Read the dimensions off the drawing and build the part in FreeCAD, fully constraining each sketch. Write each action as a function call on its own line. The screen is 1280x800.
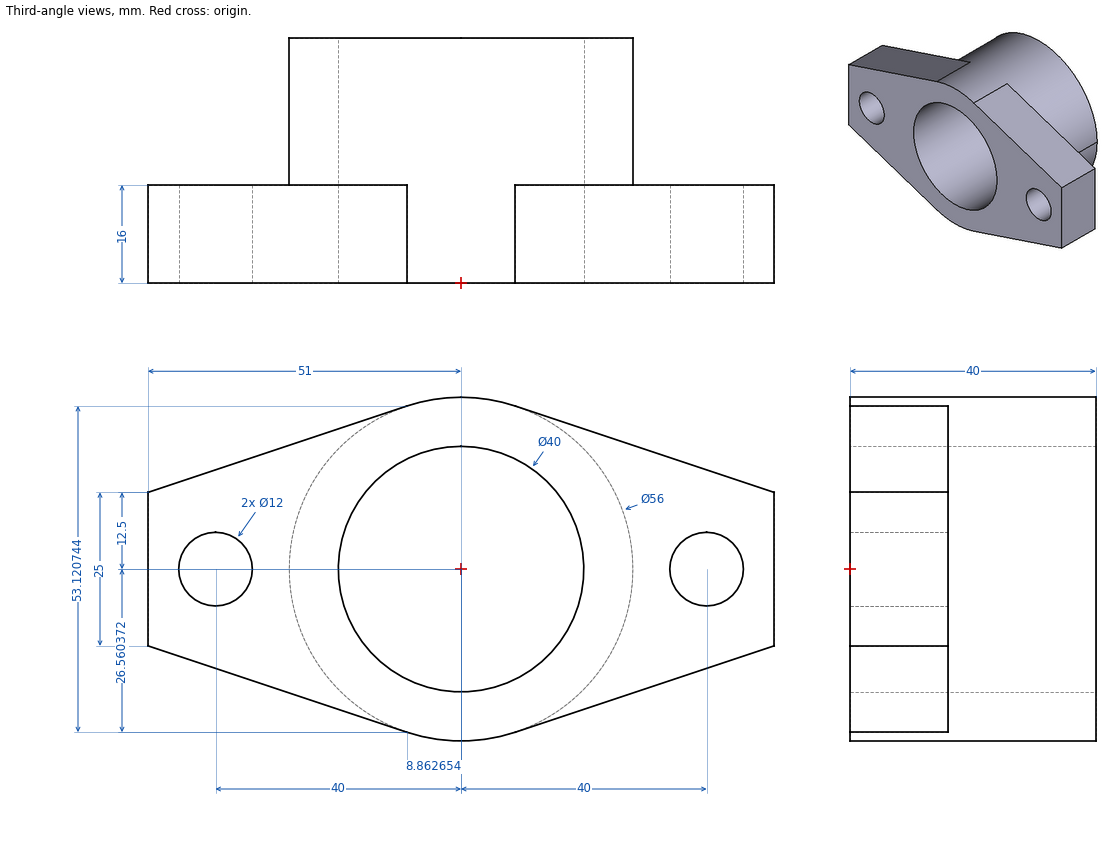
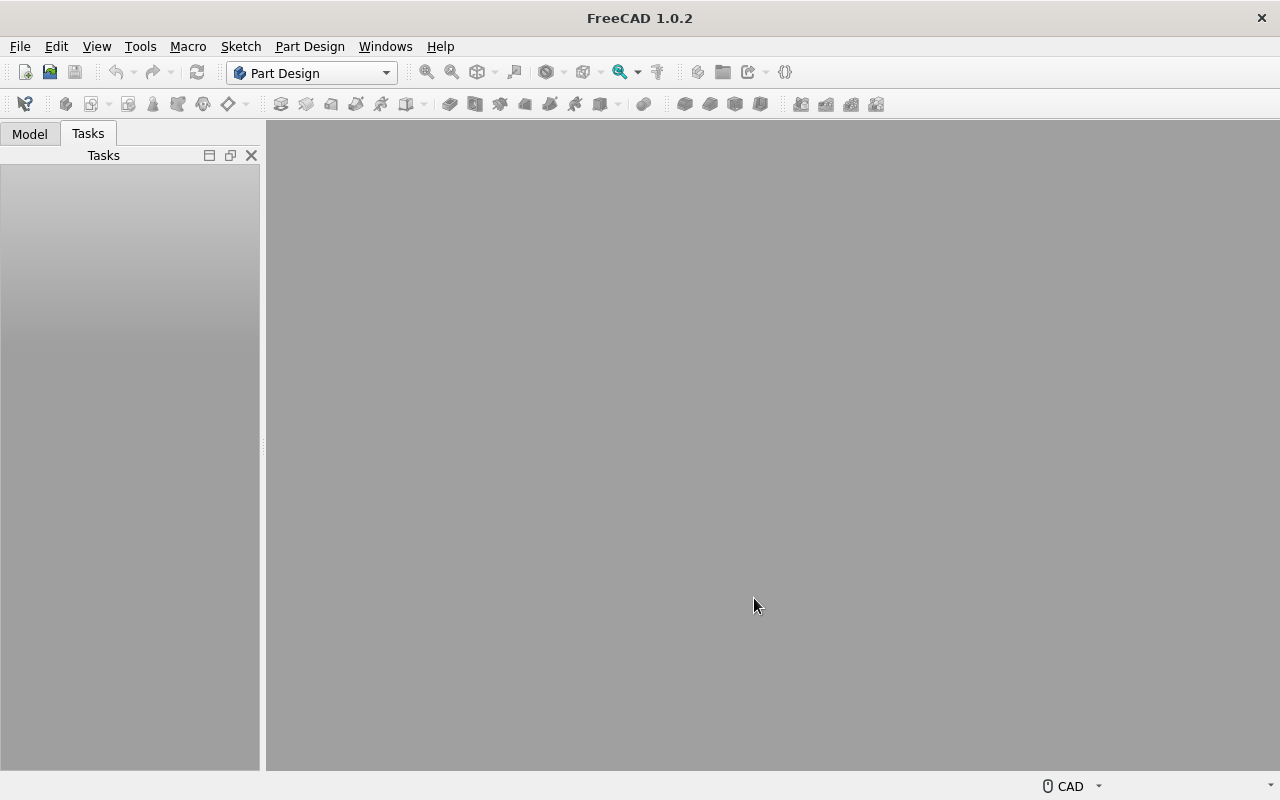
click(25, 72)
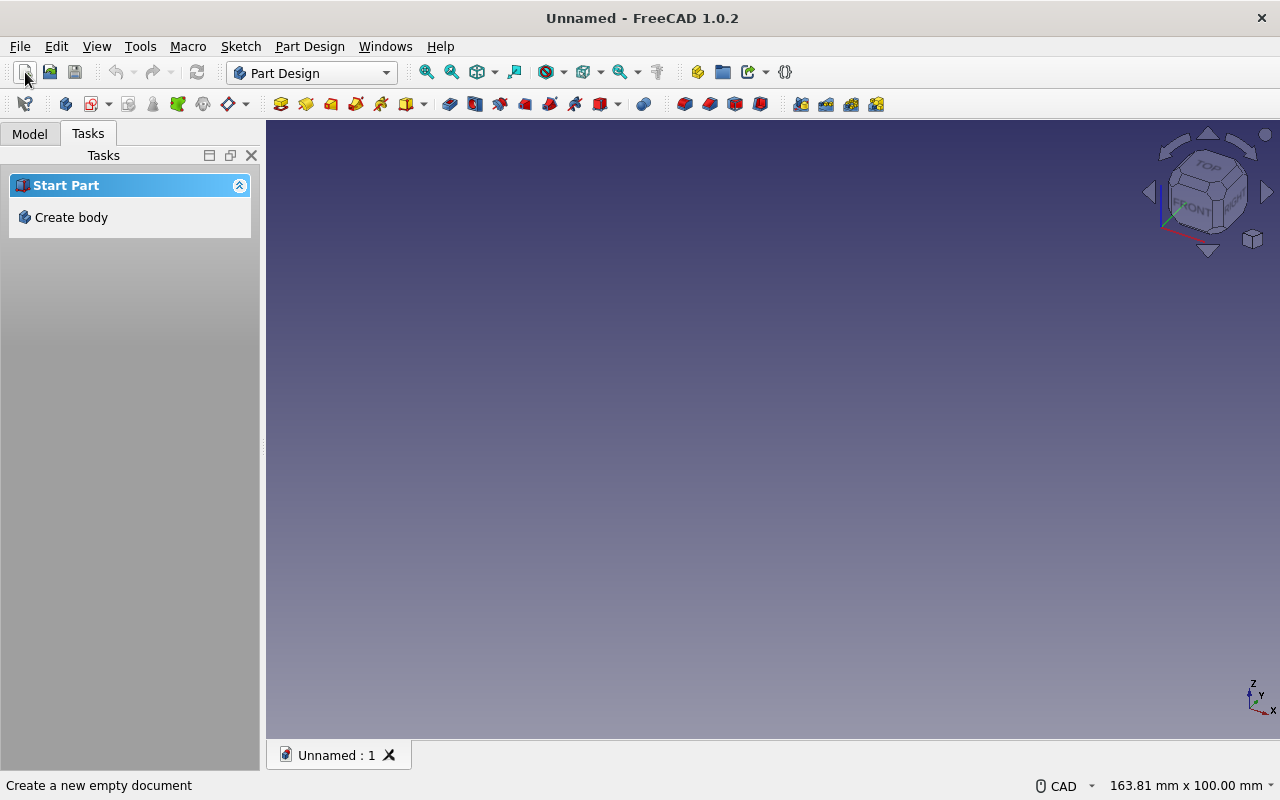
click(90, 104)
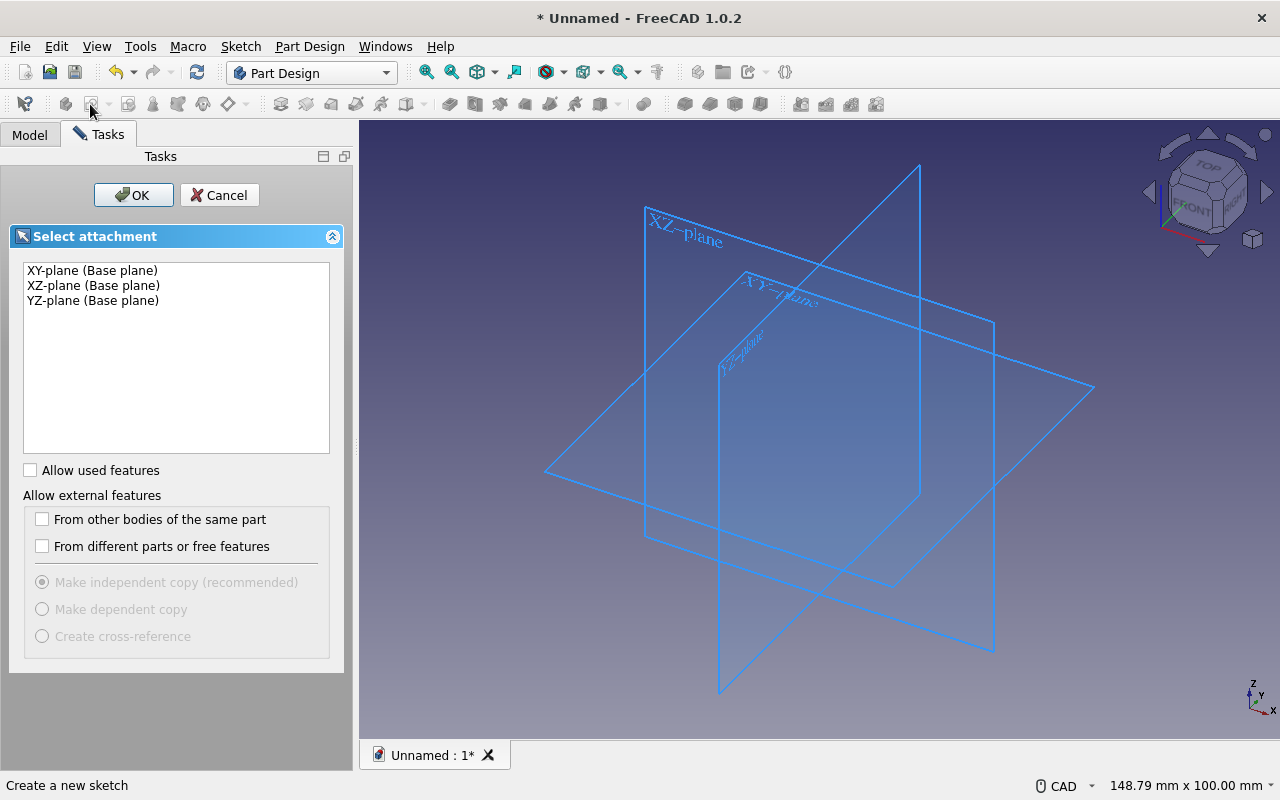
click(84, 286)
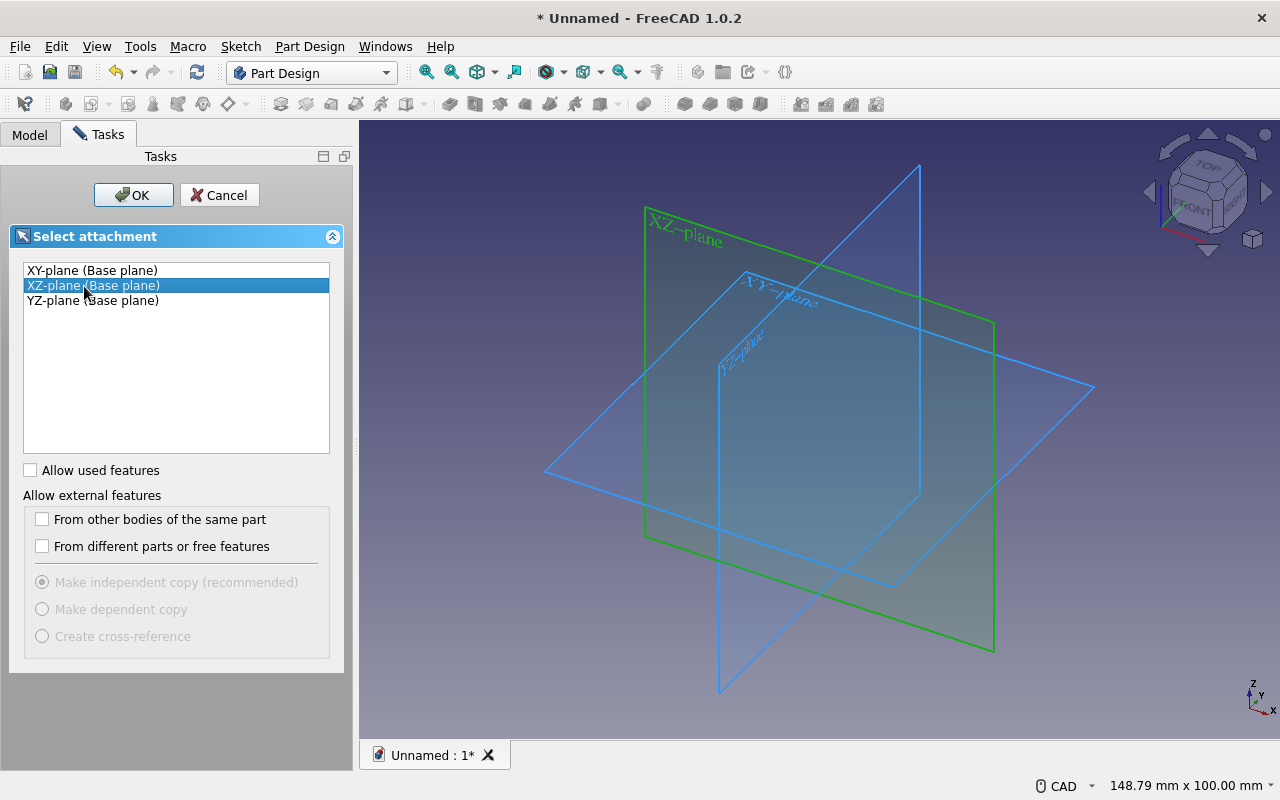
click(134, 195)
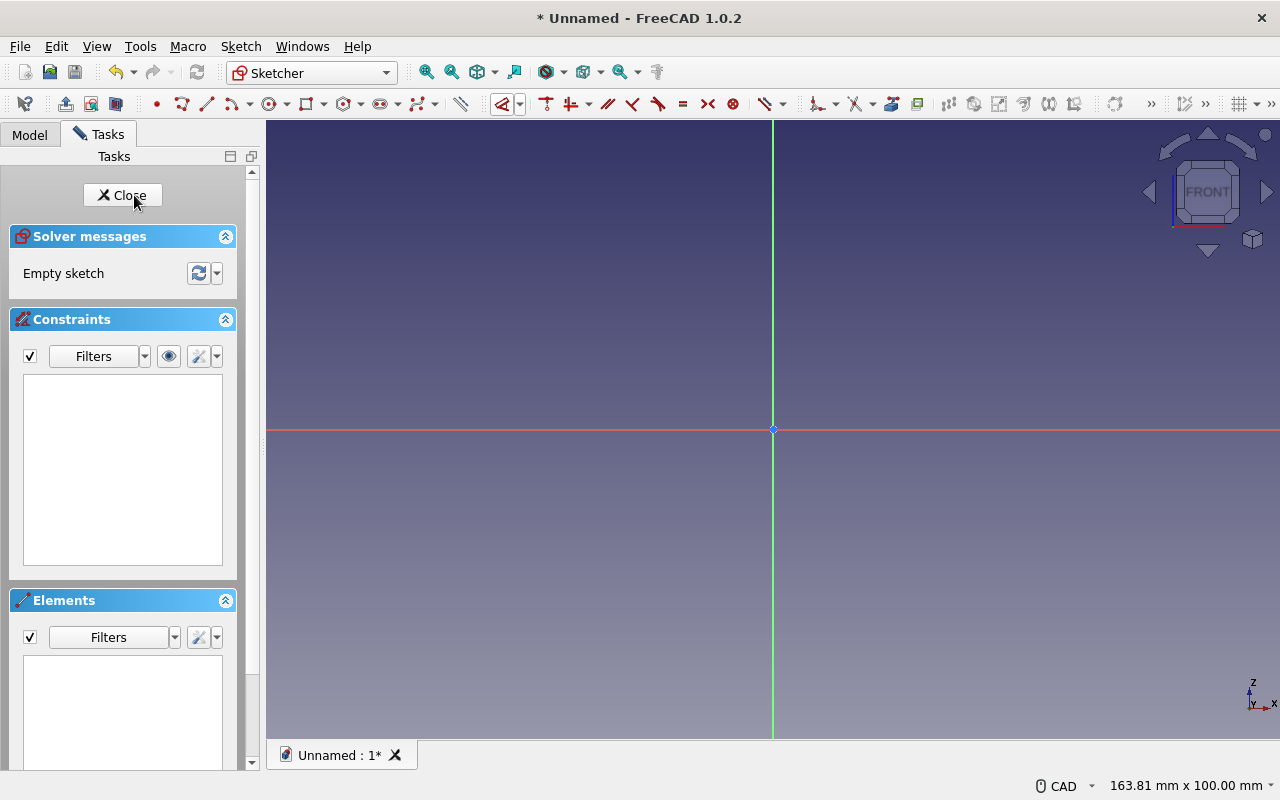
click(268, 104)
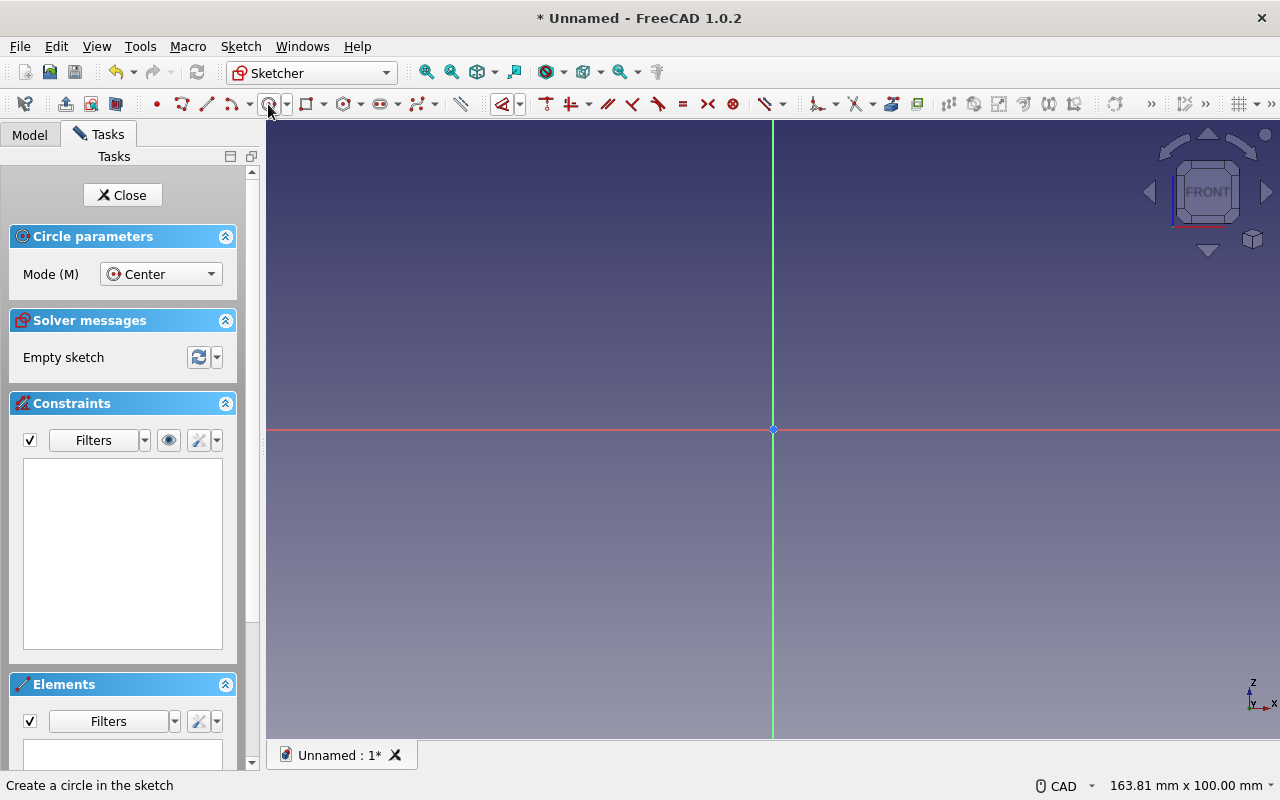
click(773, 430)
move(896, 307)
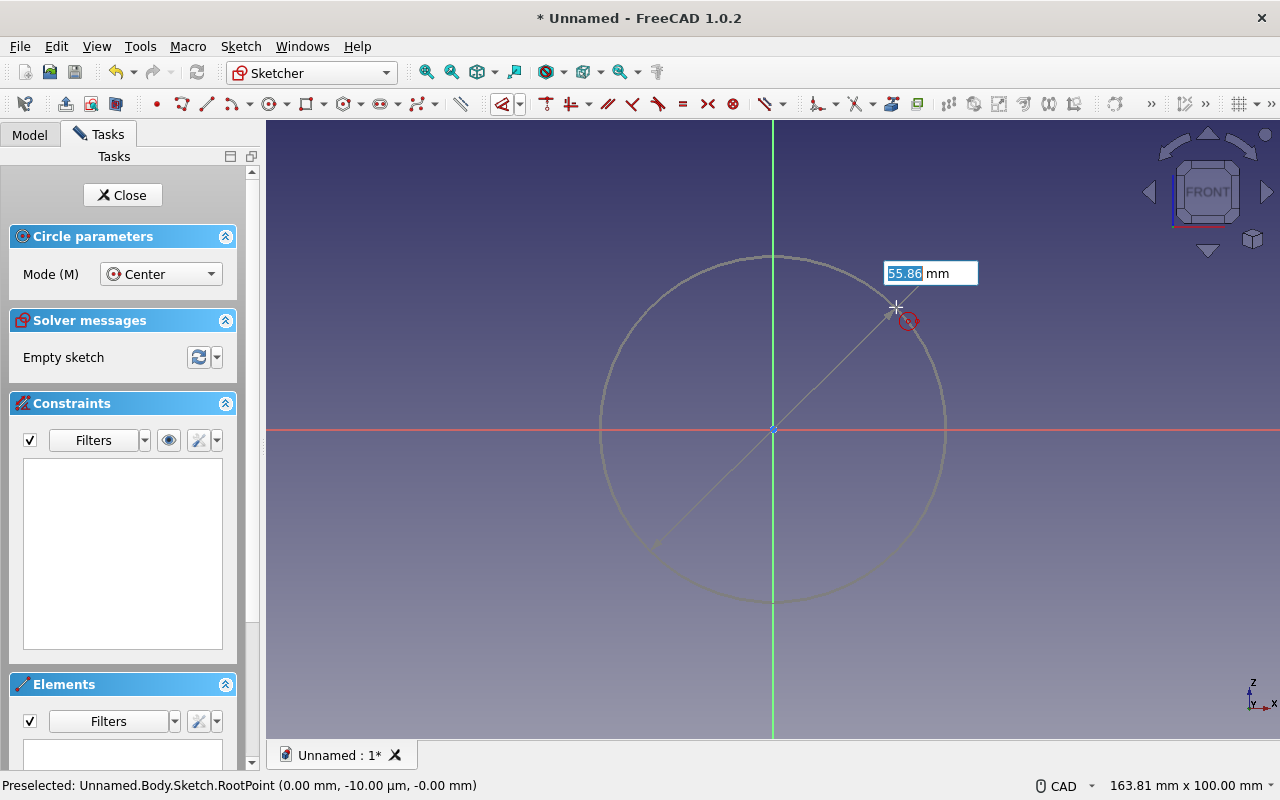
text(56)
key(Return)
key(Escape)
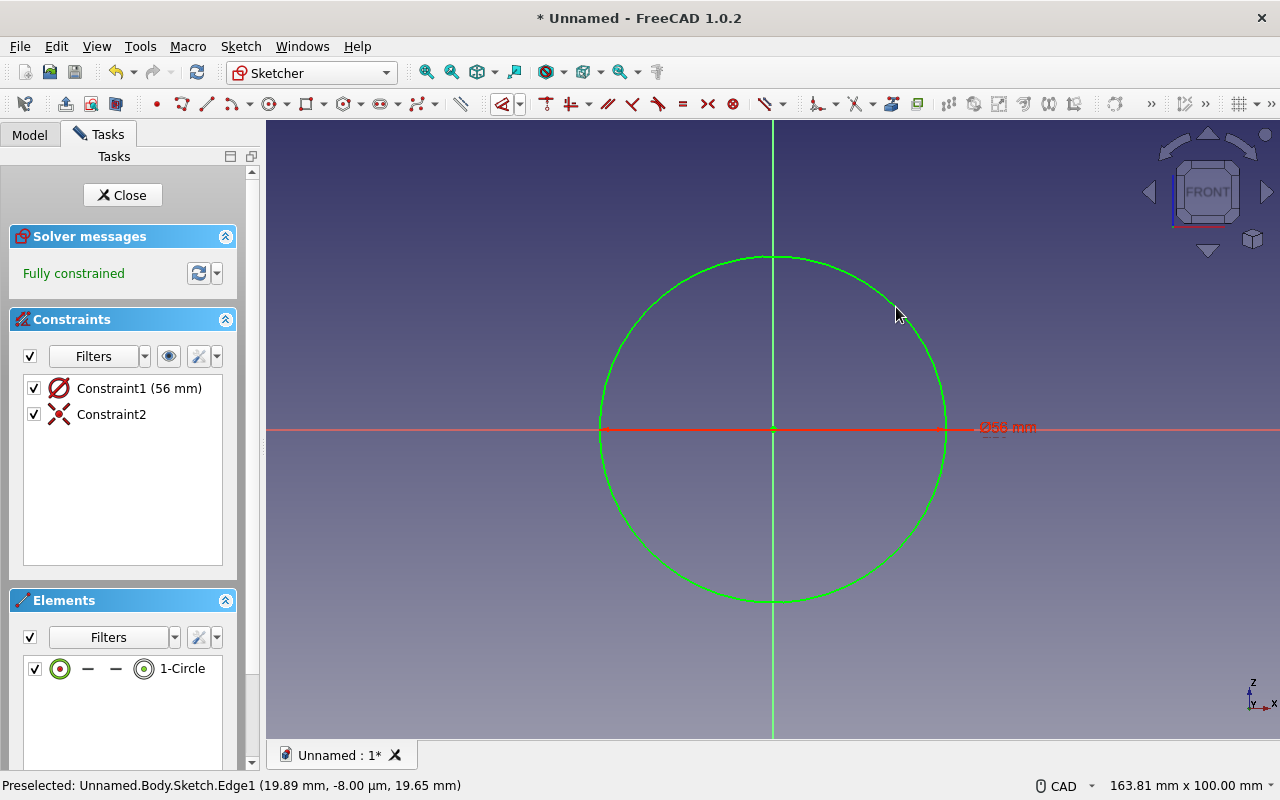
click(123, 195)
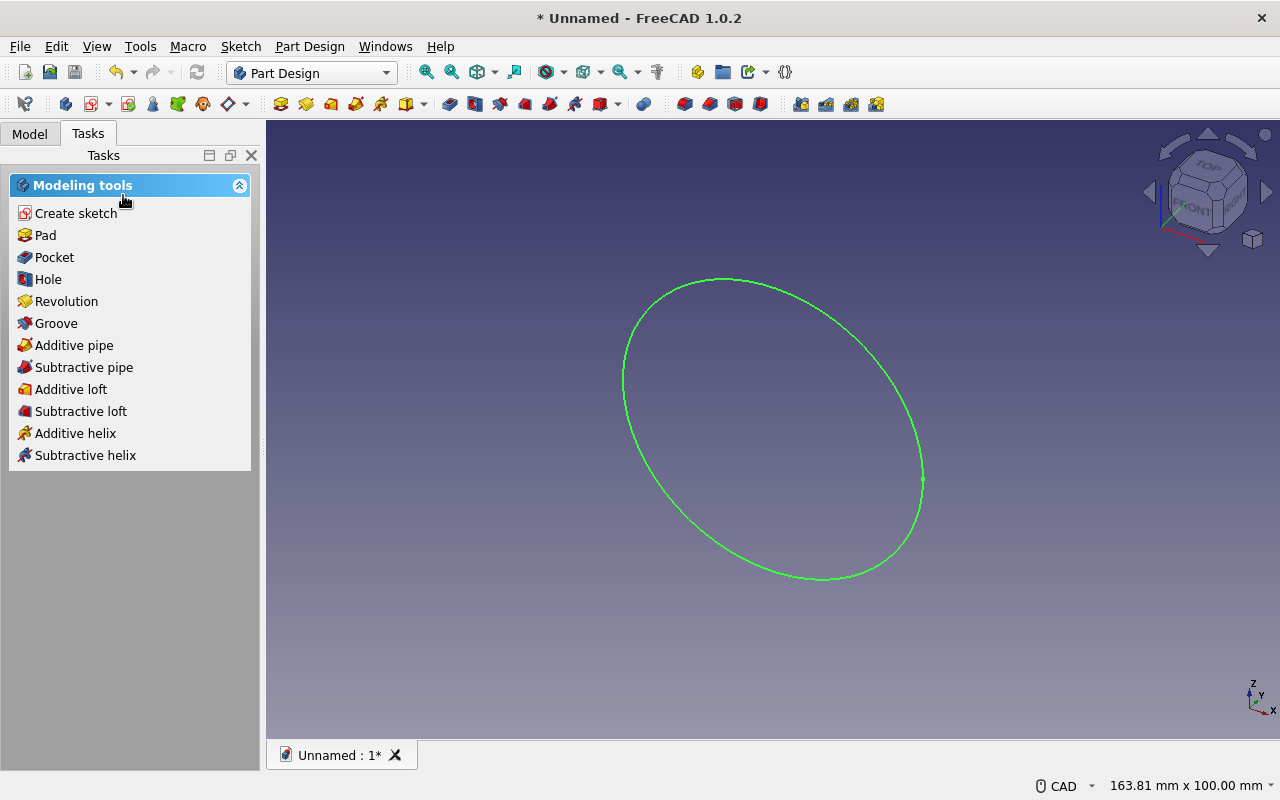
click(281, 104)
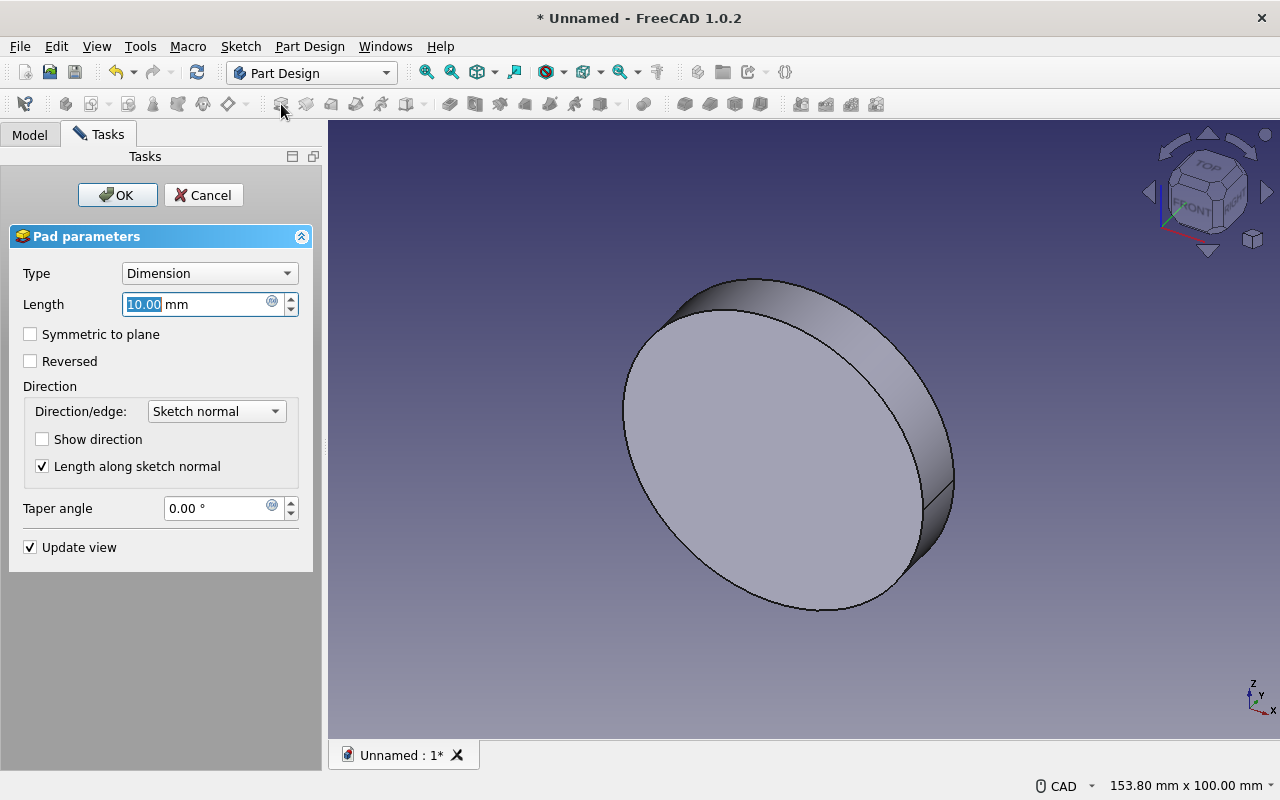
text(40)
key(Tab)